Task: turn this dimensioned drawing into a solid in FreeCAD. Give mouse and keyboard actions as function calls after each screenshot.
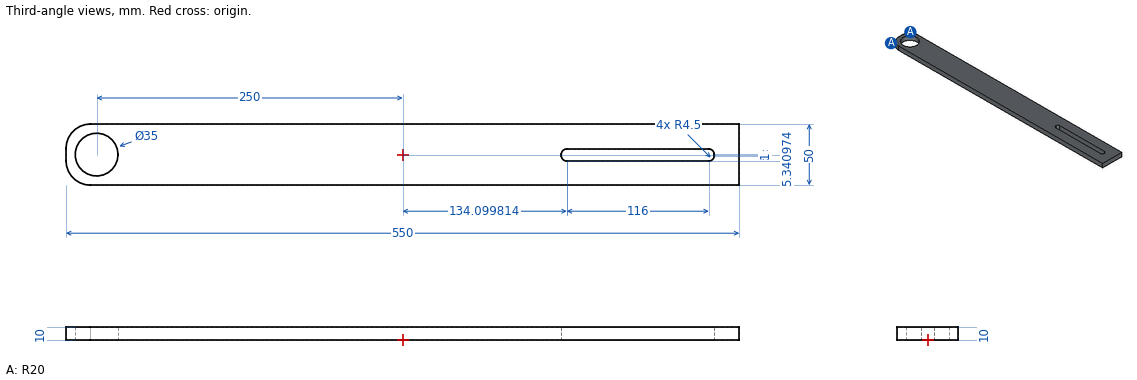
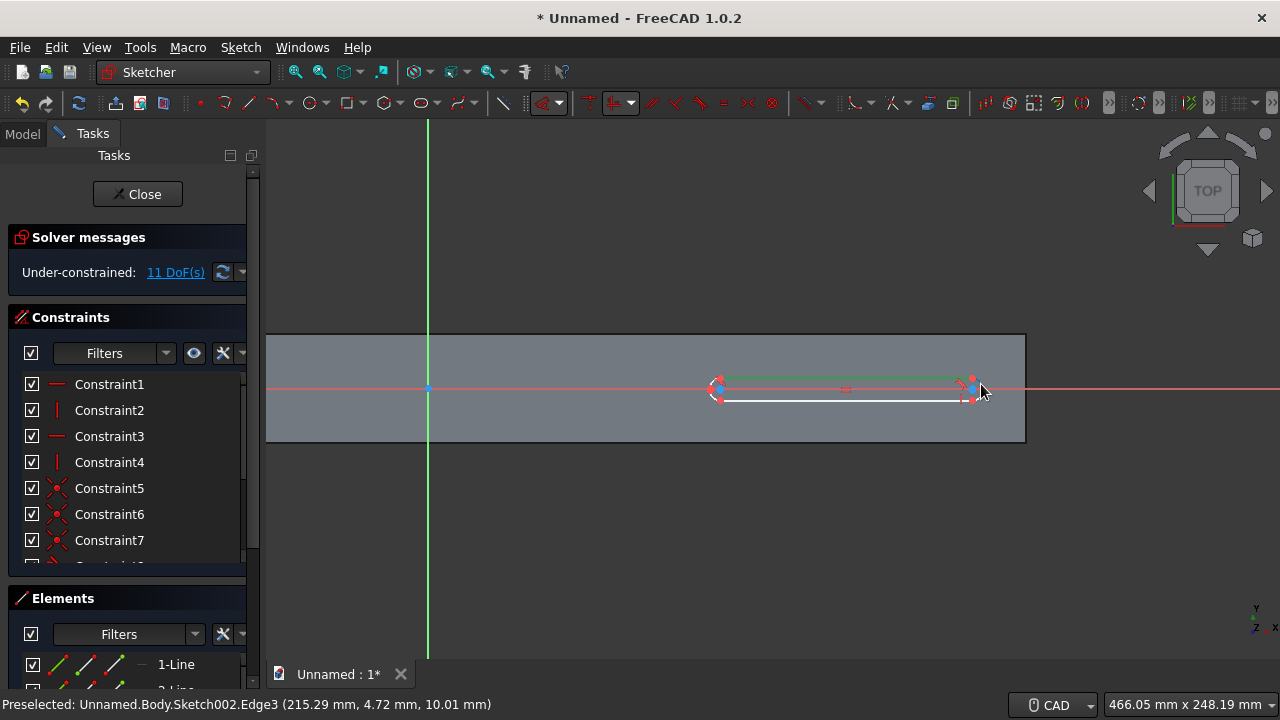
scroll(716, 379, up, 6)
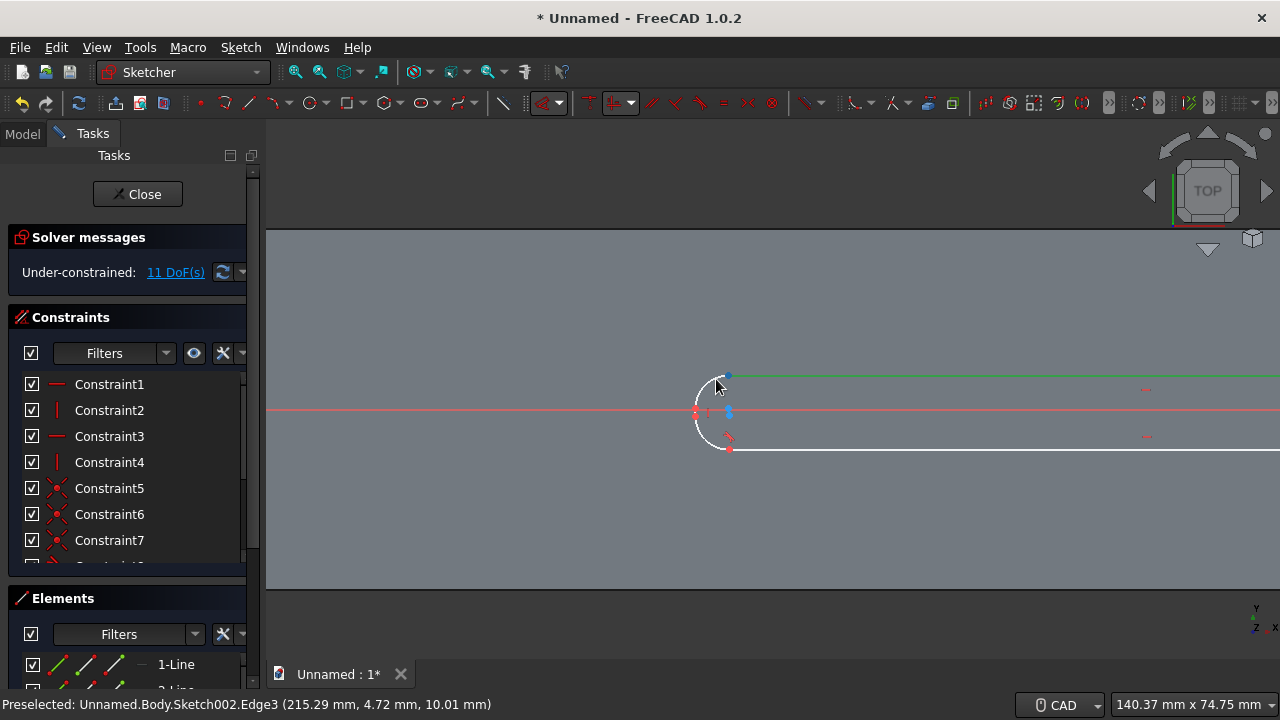
click(714, 379)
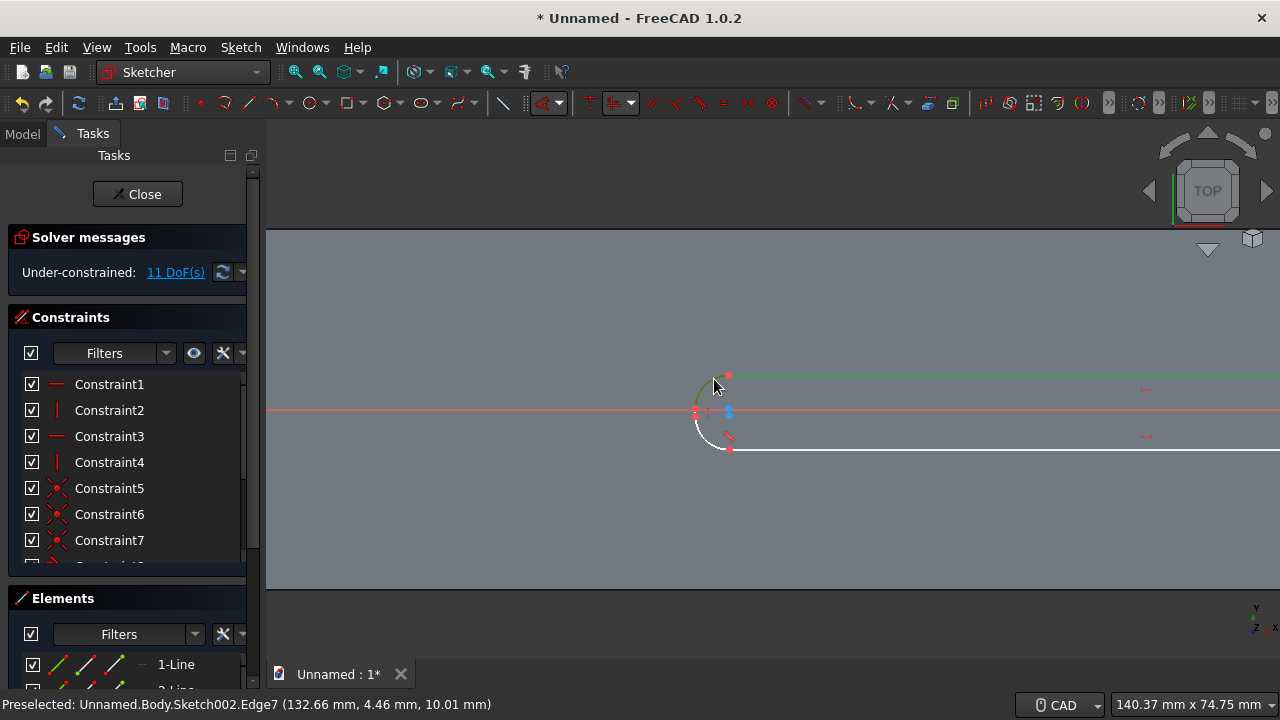
click(700, 104)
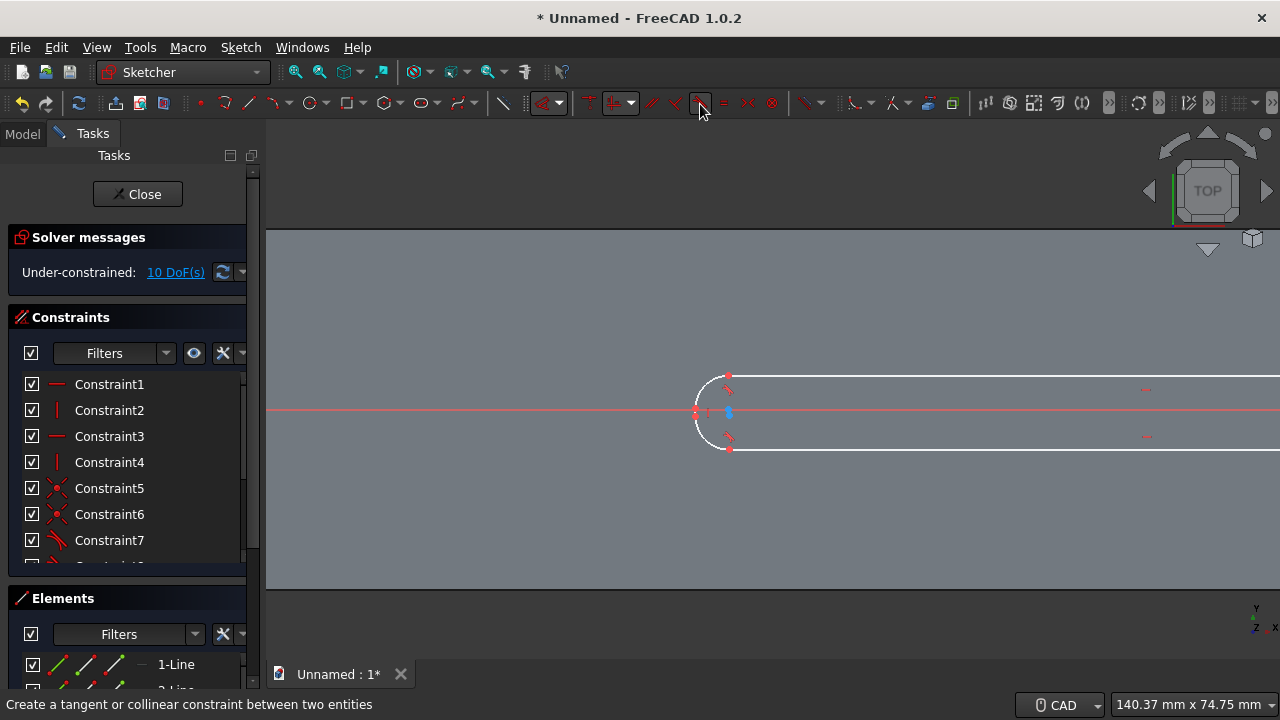
scroll(695, 413, up, 7)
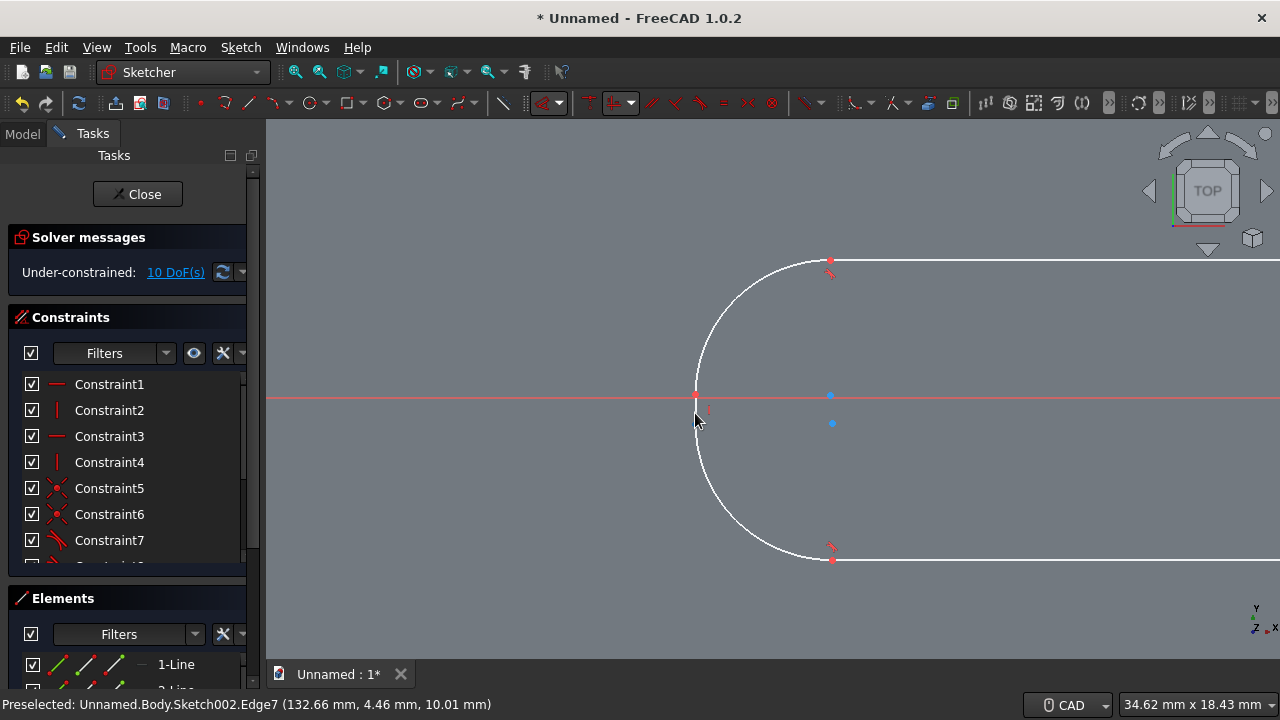
click(696, 409)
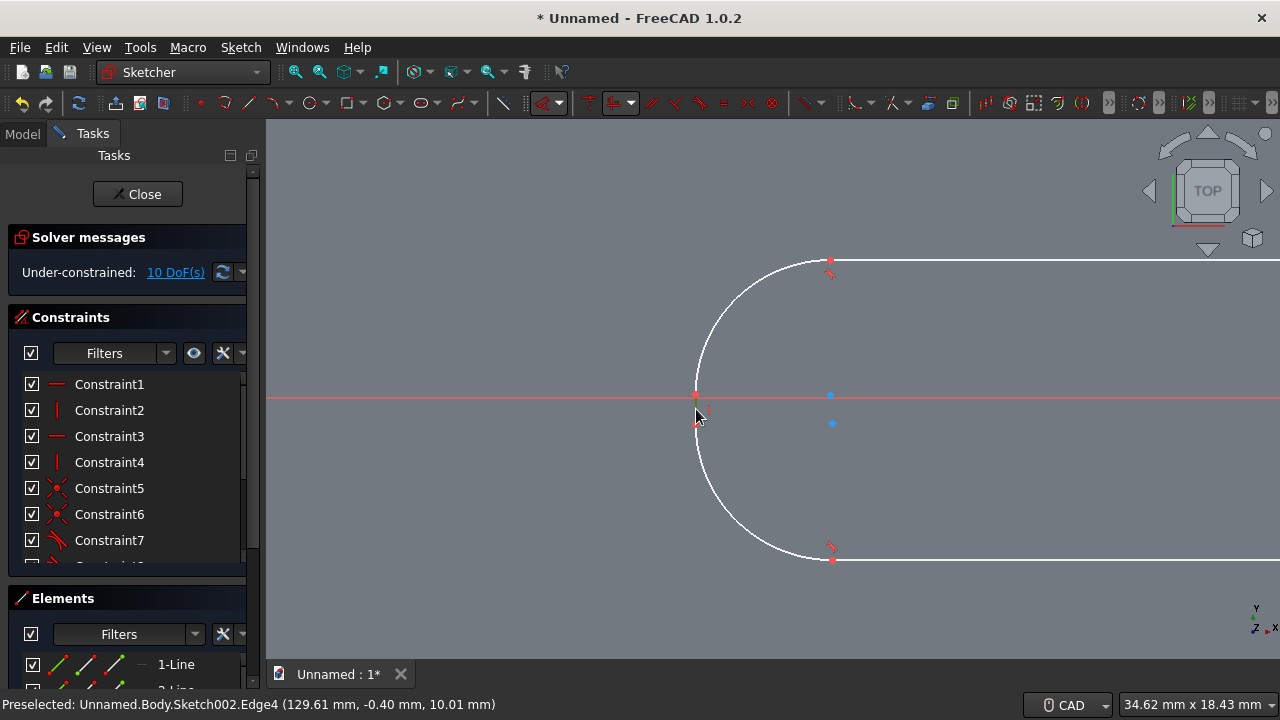
scroll(711, 387, down, 13)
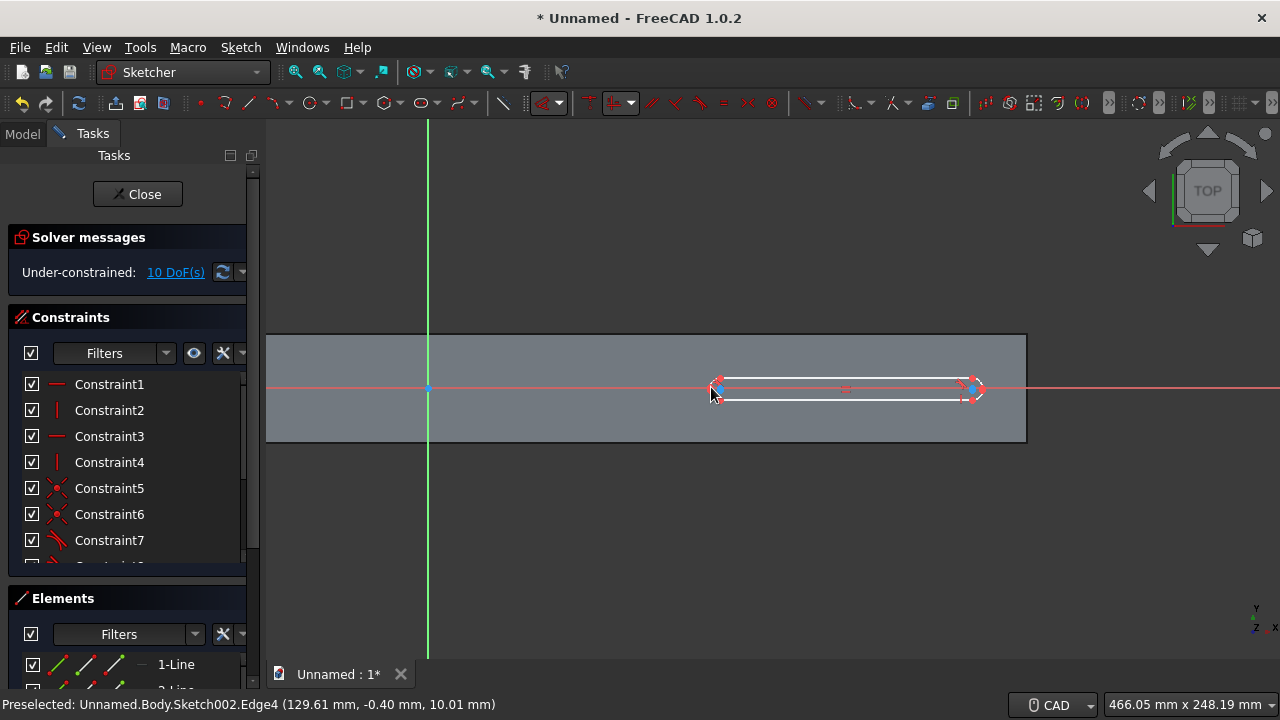
scroll(716, 379, up, 6)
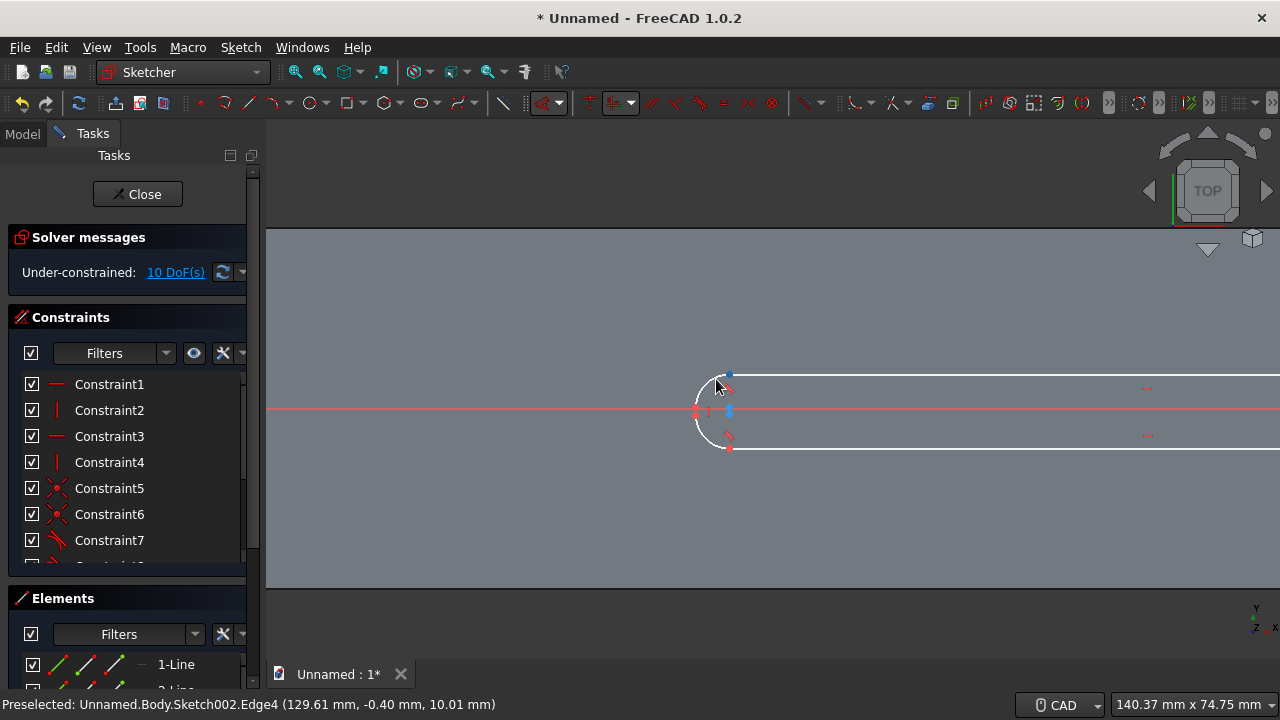
click(714, 378)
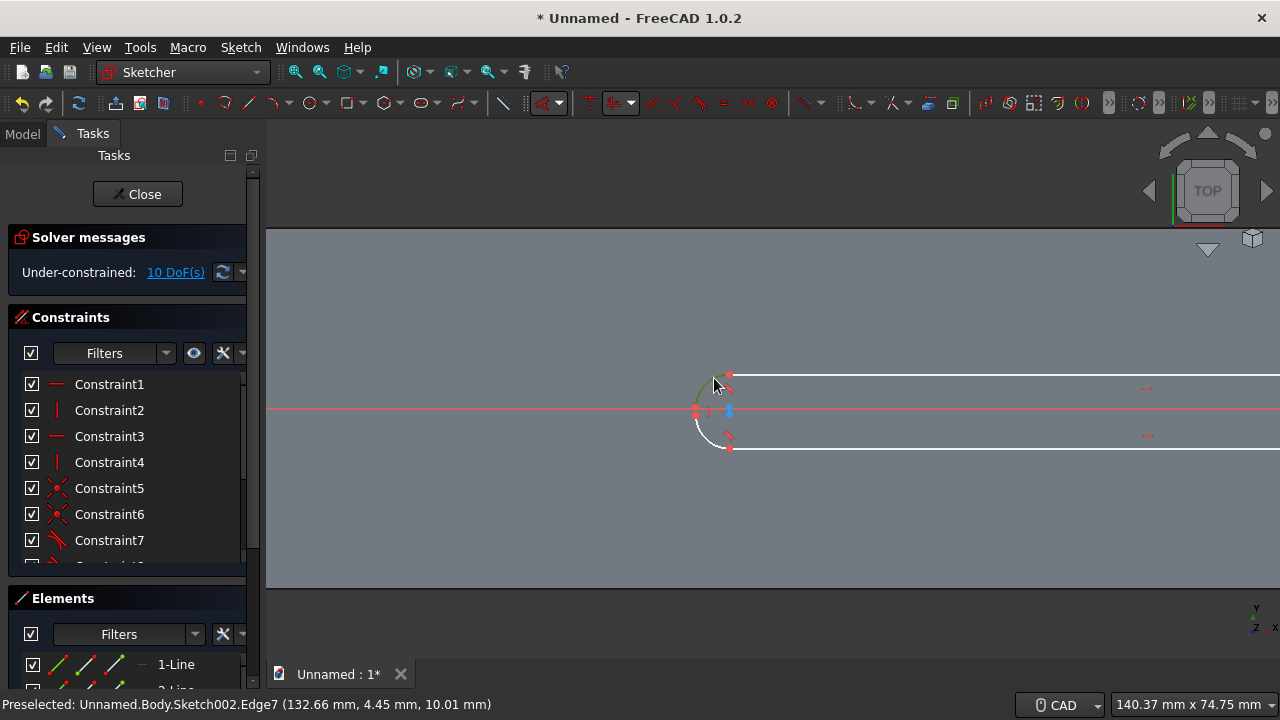
click(700, 104)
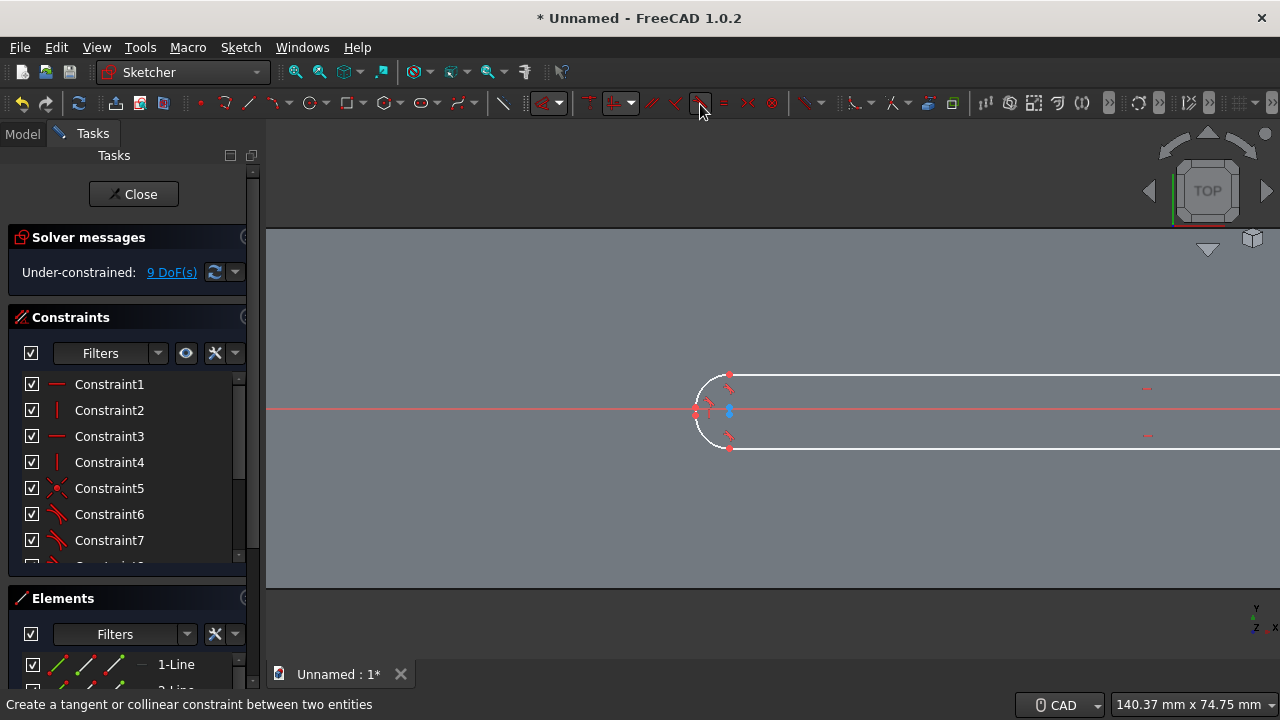
scroll(696, 412, up, 7)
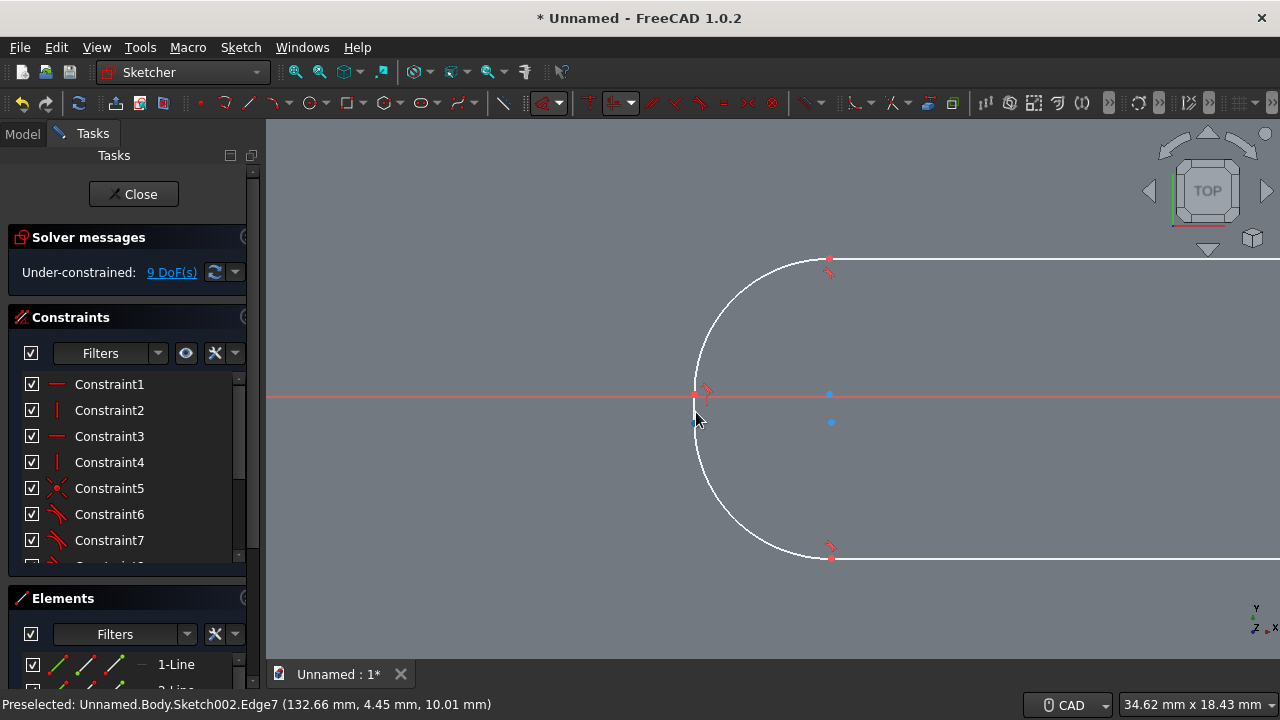
click(694, 409)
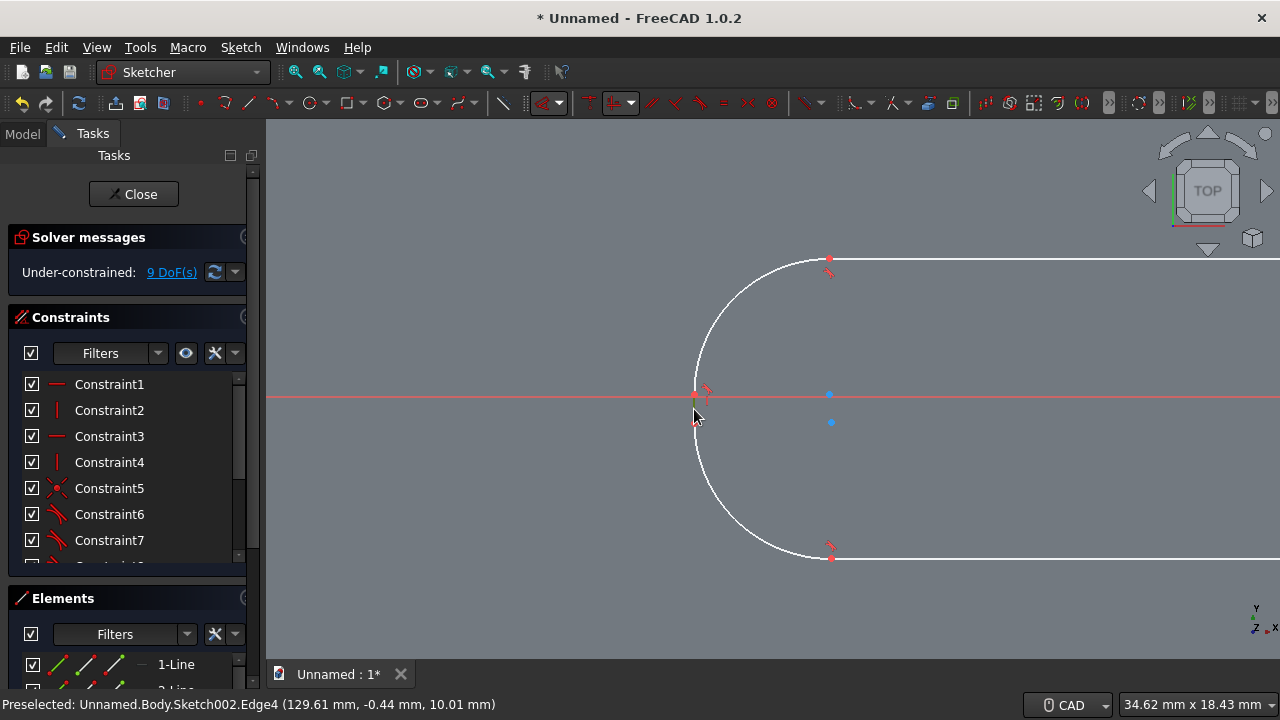
scroll(711, 388, down, 13)